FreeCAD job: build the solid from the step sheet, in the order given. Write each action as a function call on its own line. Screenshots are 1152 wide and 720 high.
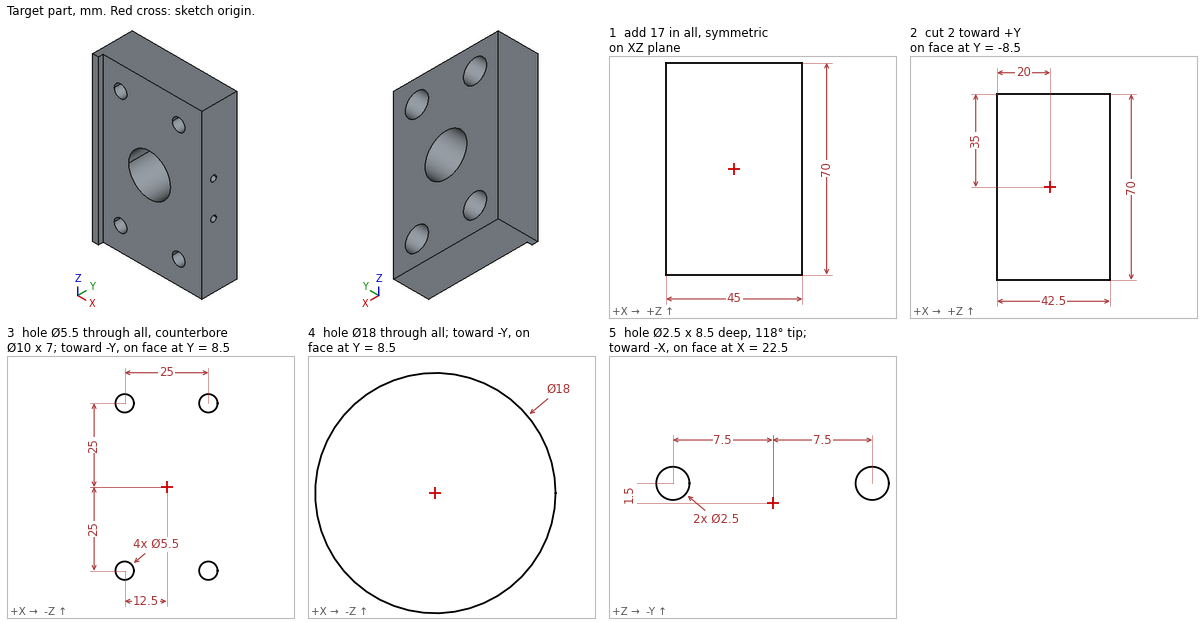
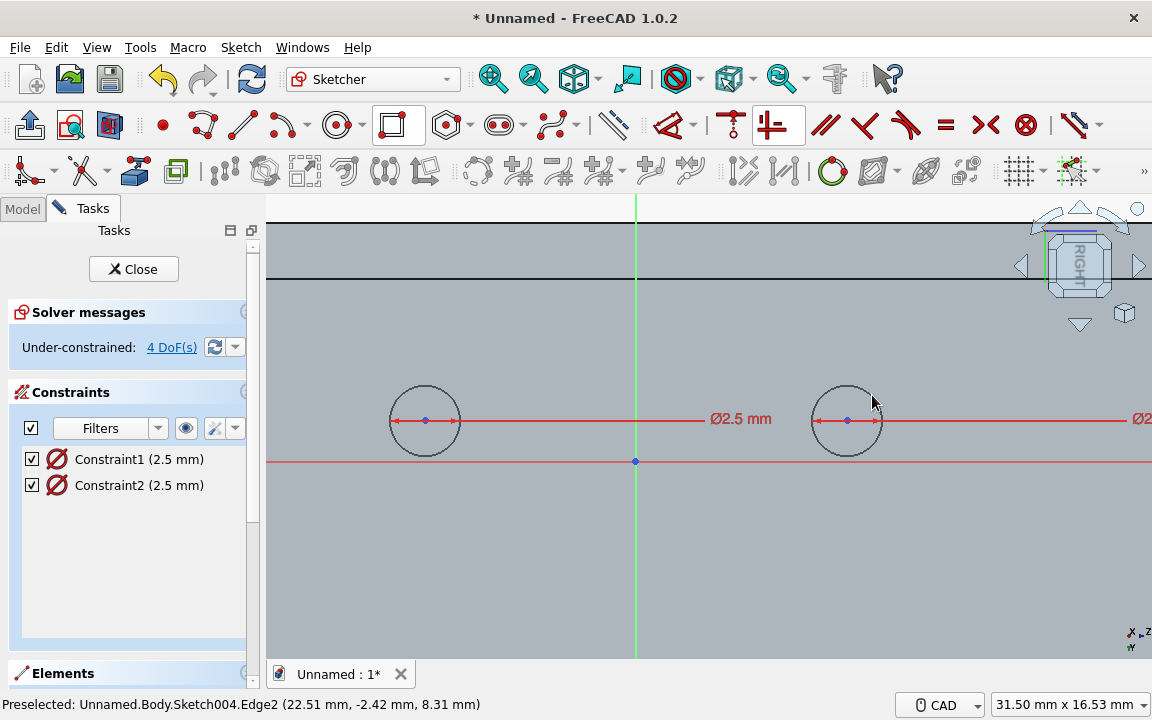
click(425, 421)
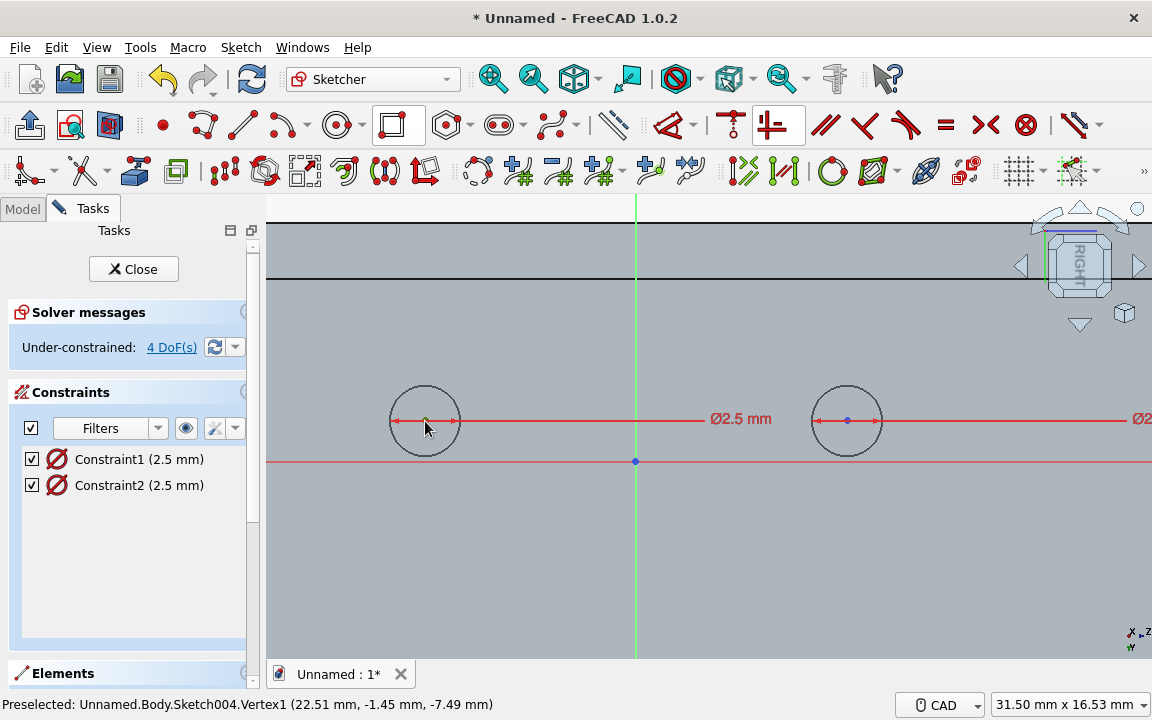
click(847, 421)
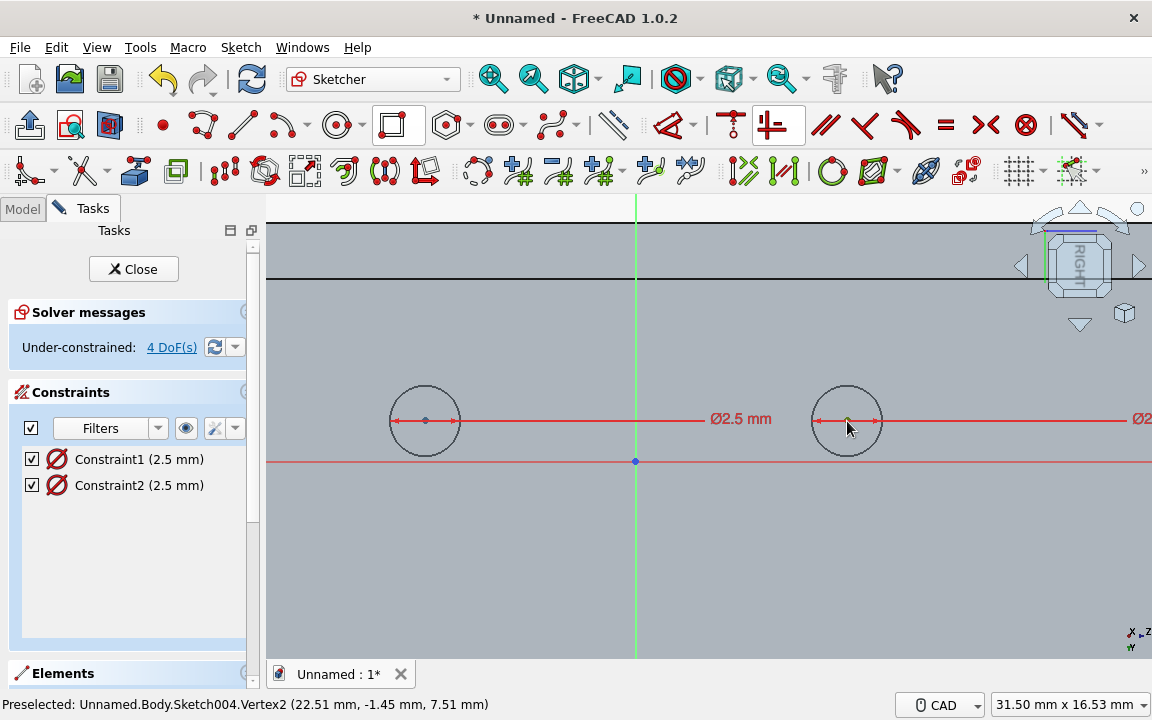
click(800, 126)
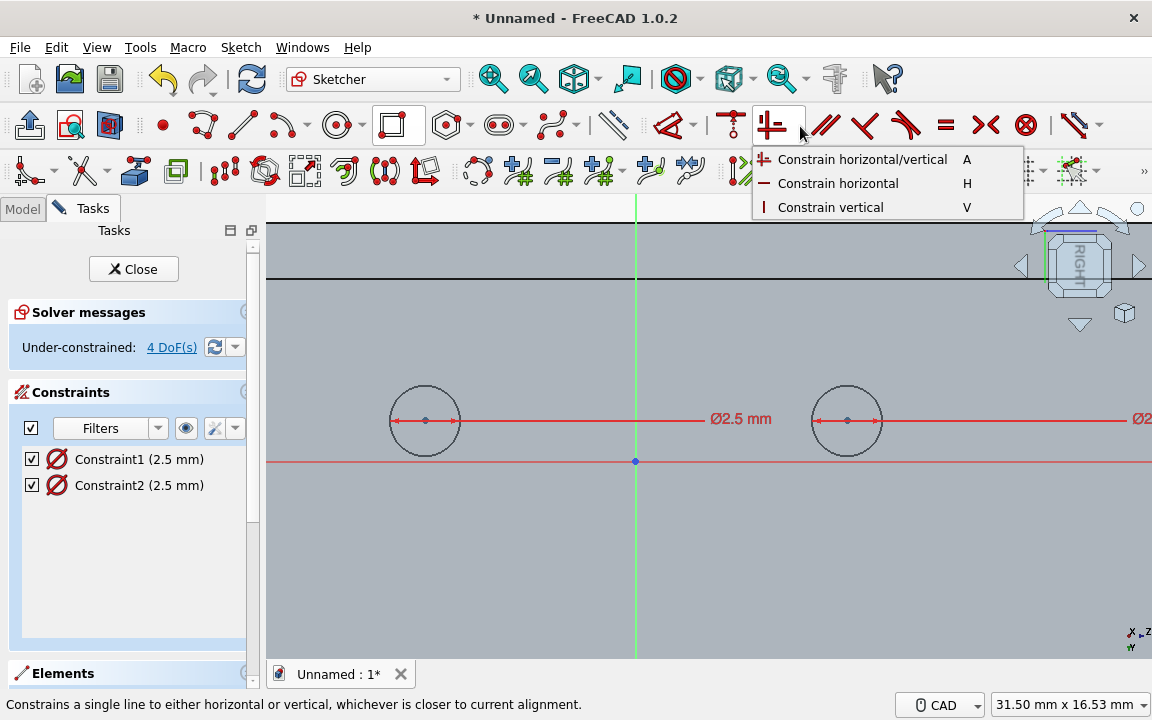
click(888, 183)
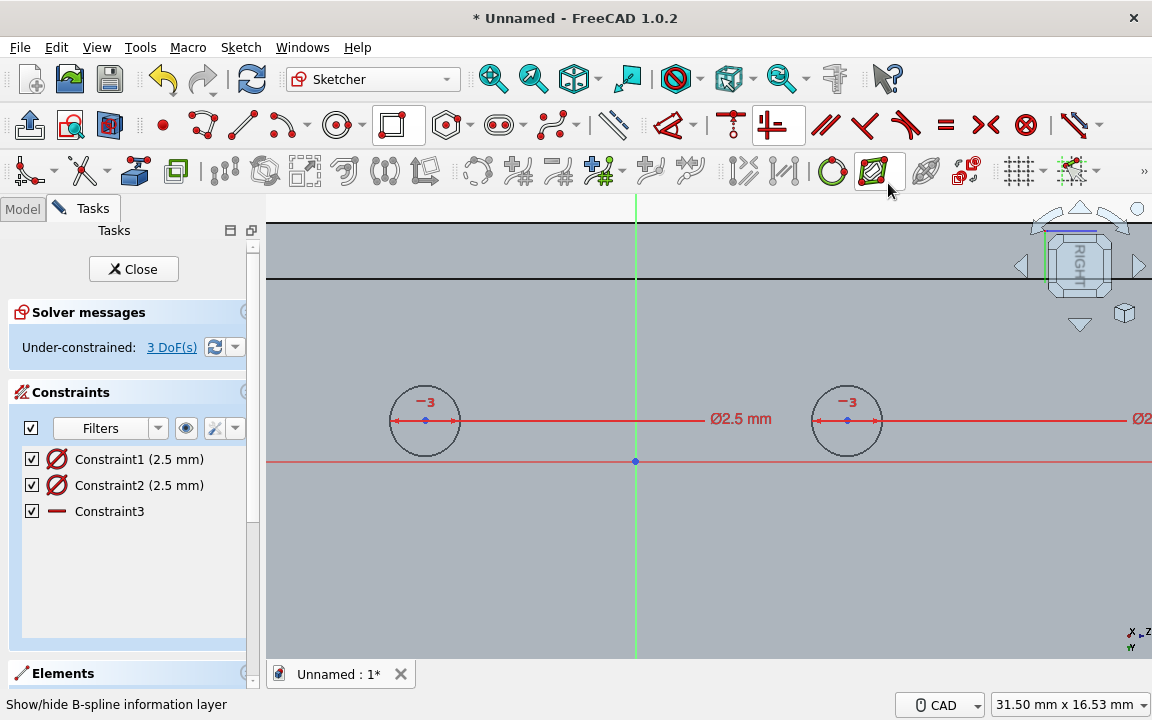
click(668, 126)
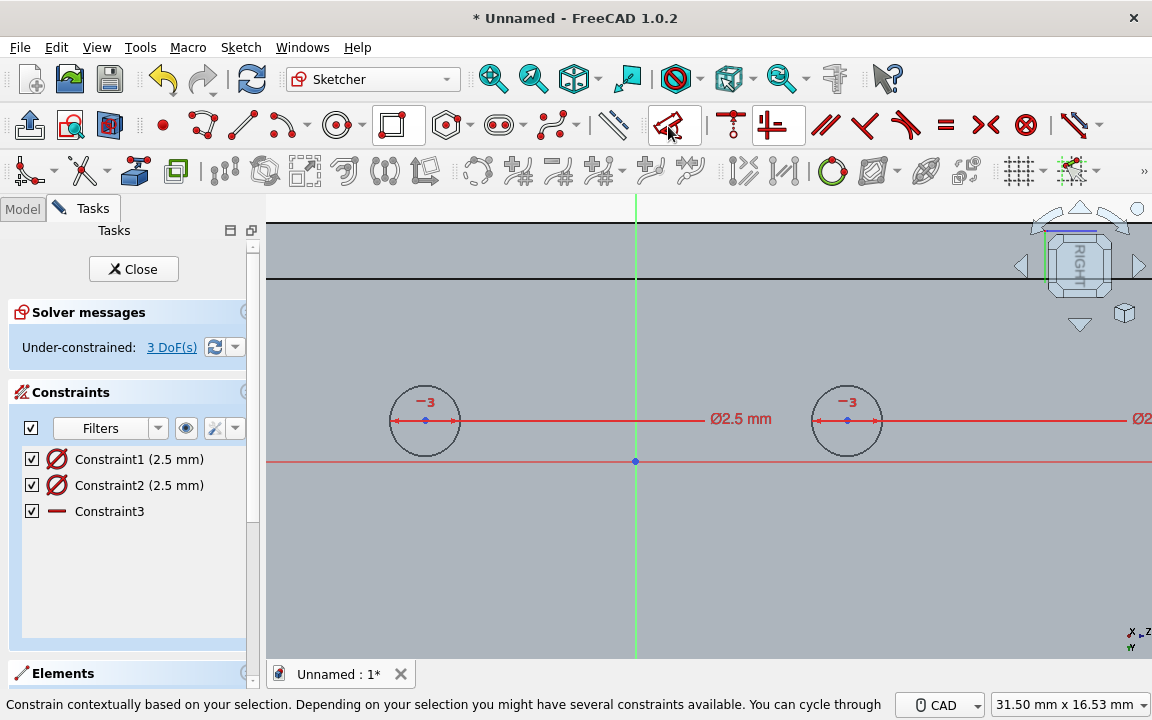
click(425, 421)
click(530, 496)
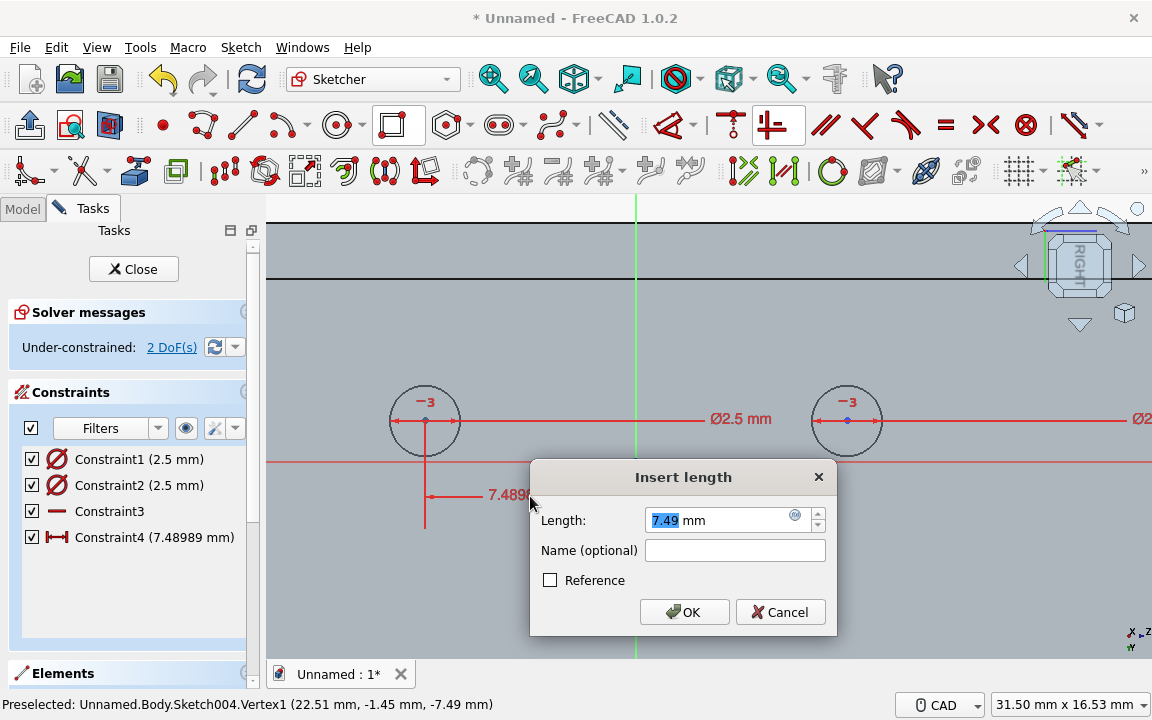
text(7.5)
key(Return)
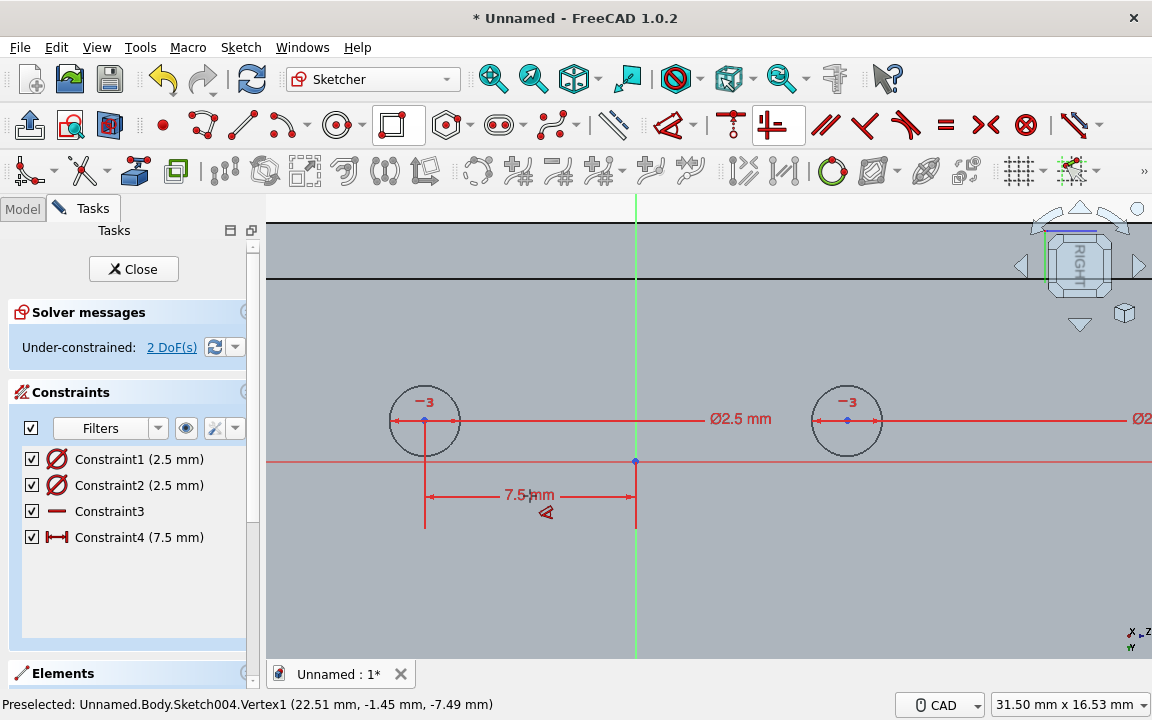
click(425, 421)
click(670, 441)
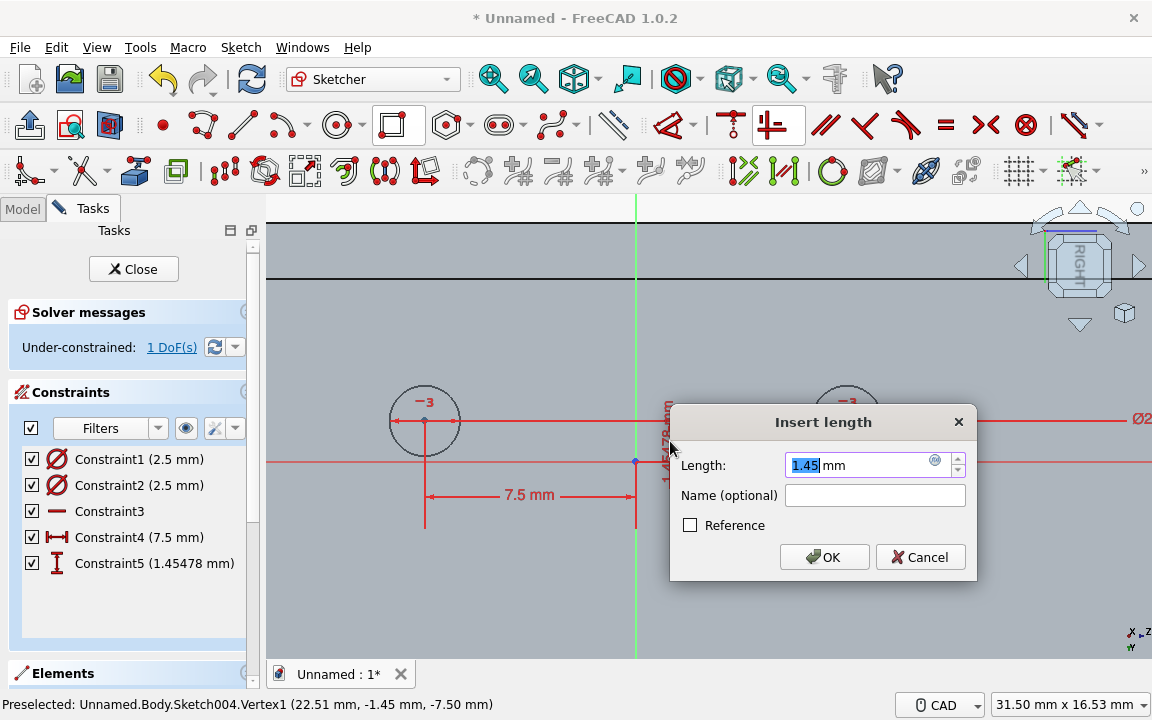
text(1.5)
key(Return)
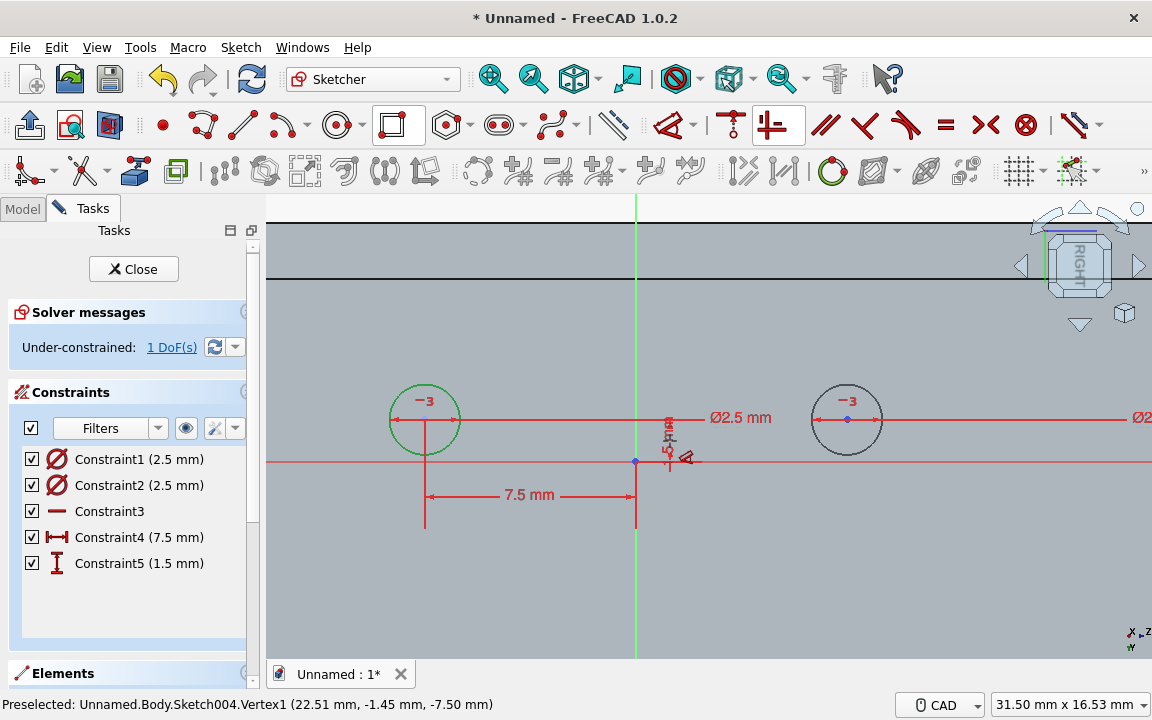
click(847, 420)
click(741, 496)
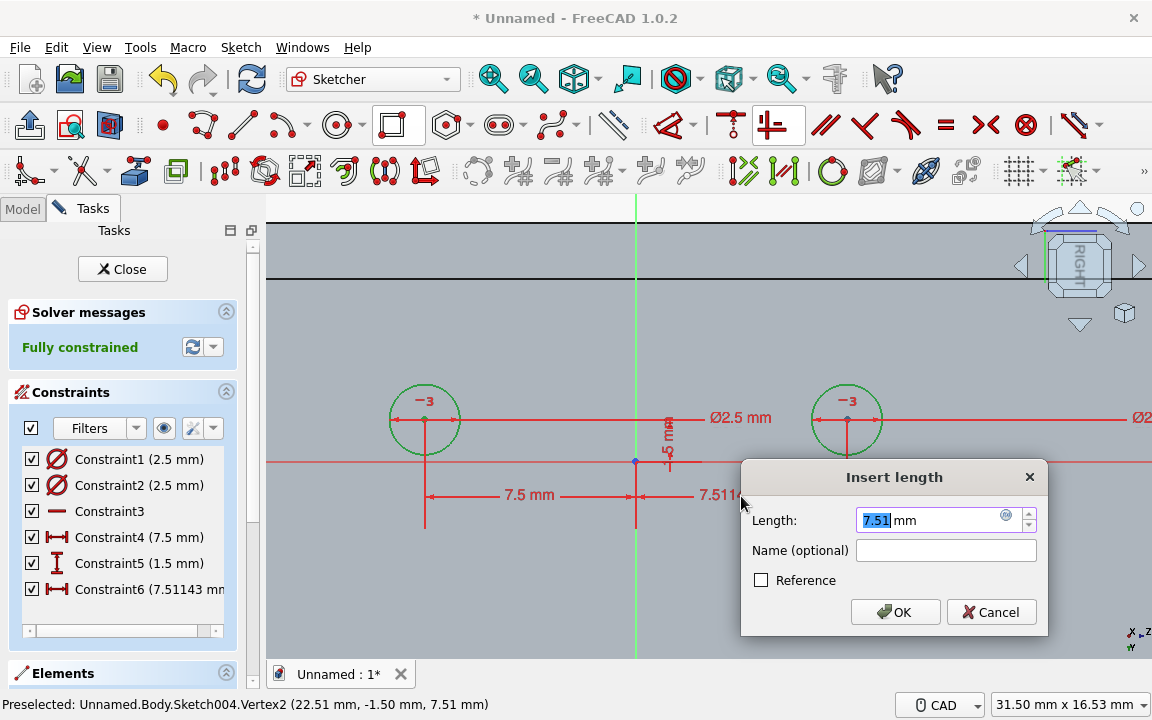
text(7.5)
key(Return)
key(Escape)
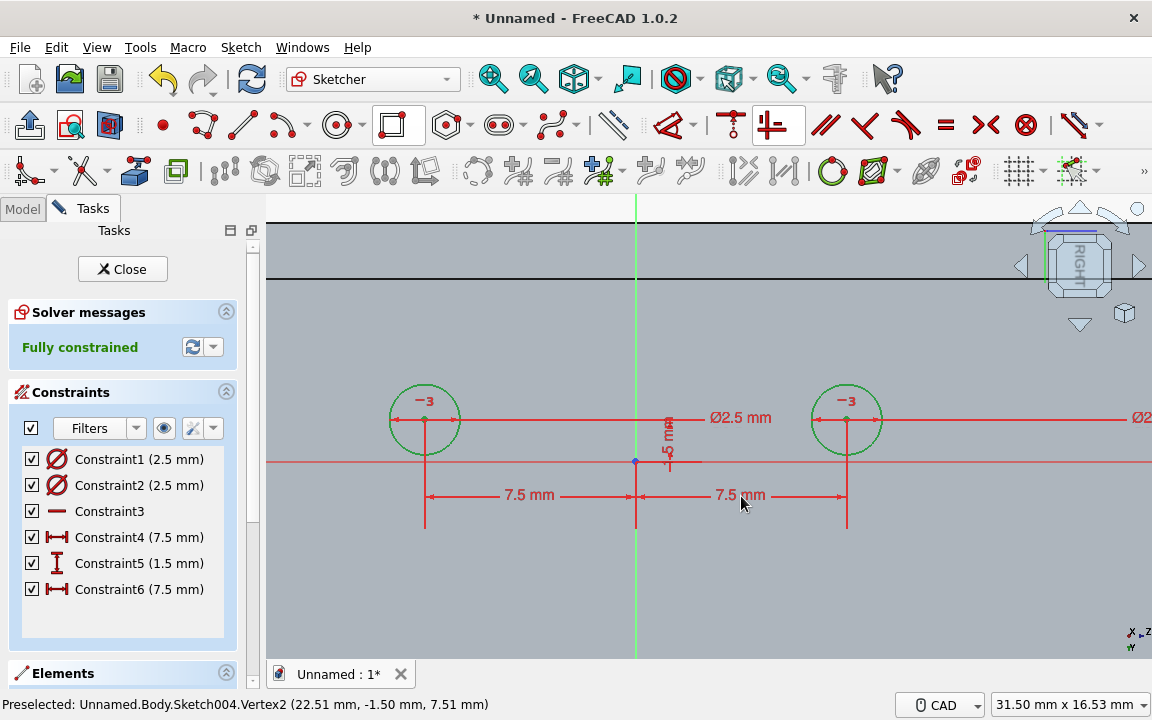
click(123, 269)